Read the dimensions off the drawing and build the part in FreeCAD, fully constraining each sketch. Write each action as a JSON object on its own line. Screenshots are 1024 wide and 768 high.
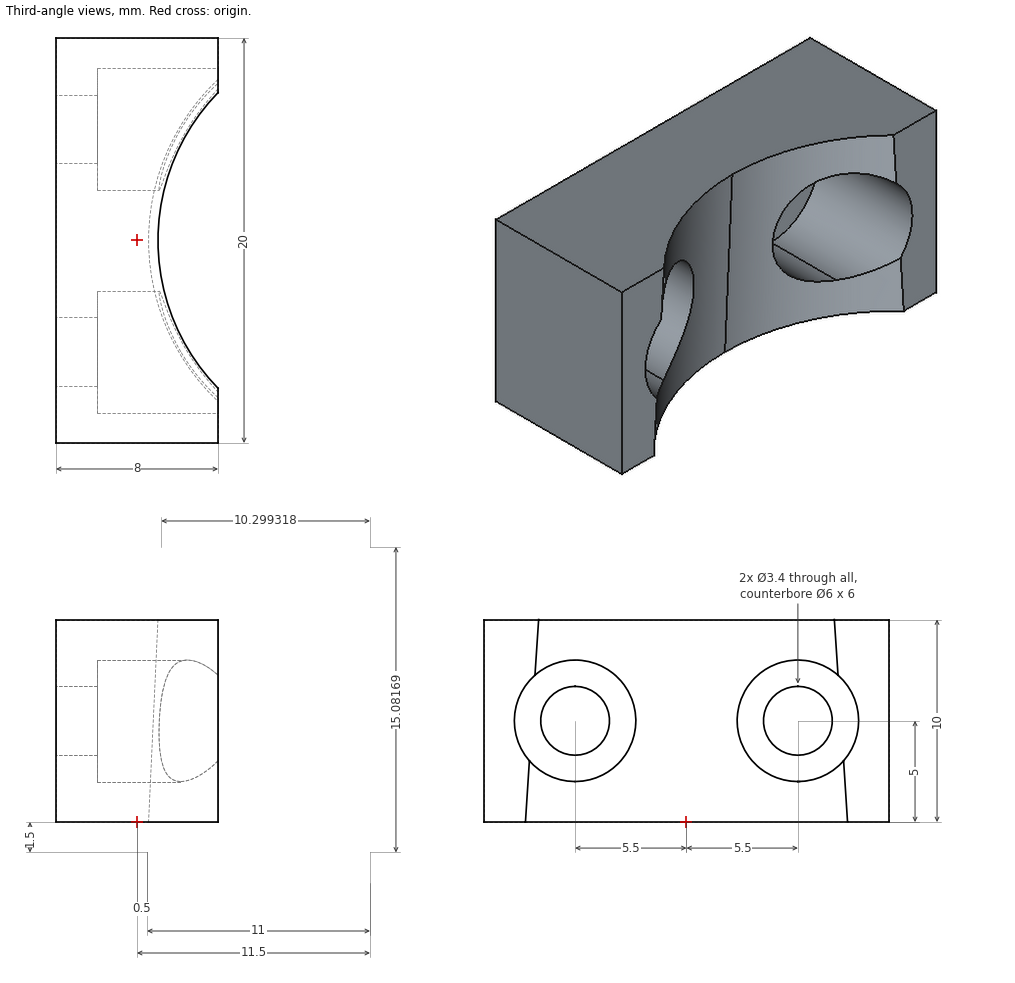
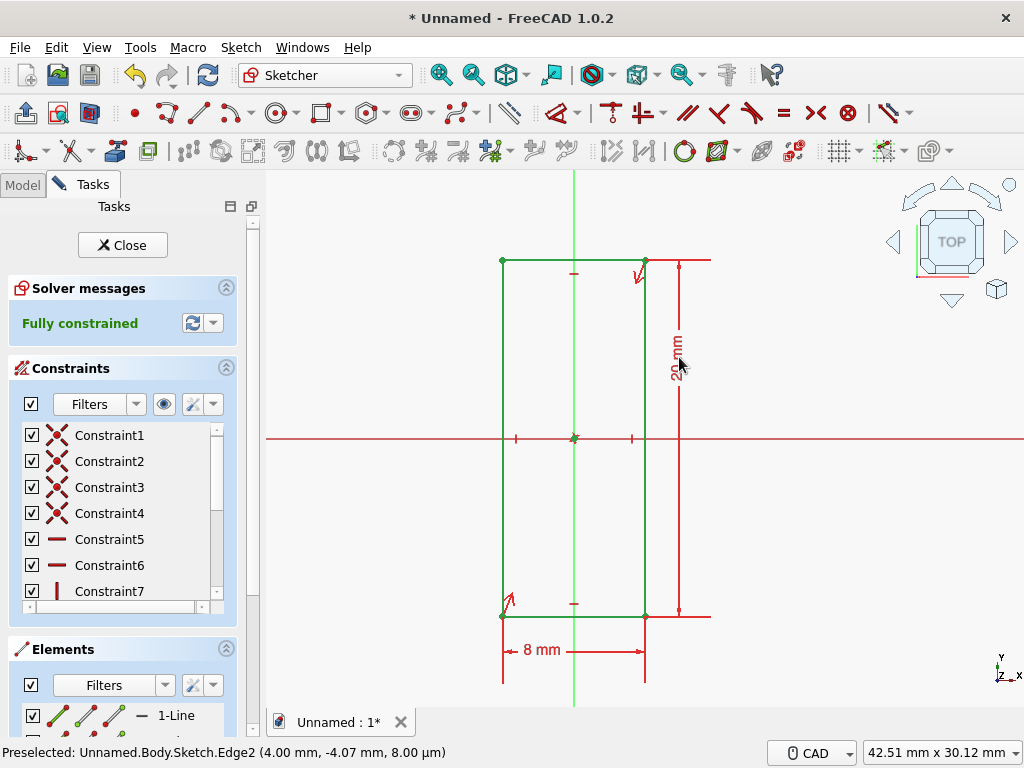
{"action": "left_click", "coordinate": [123, 245]}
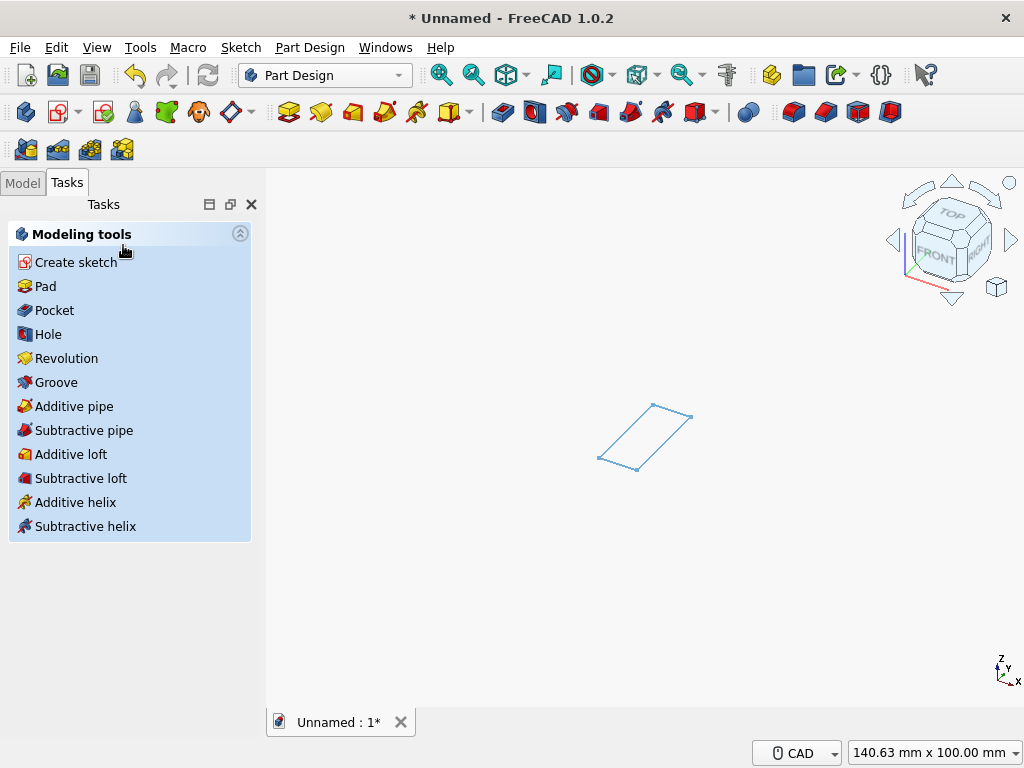
{"action": "left_click", "coordinate": [290, 112]}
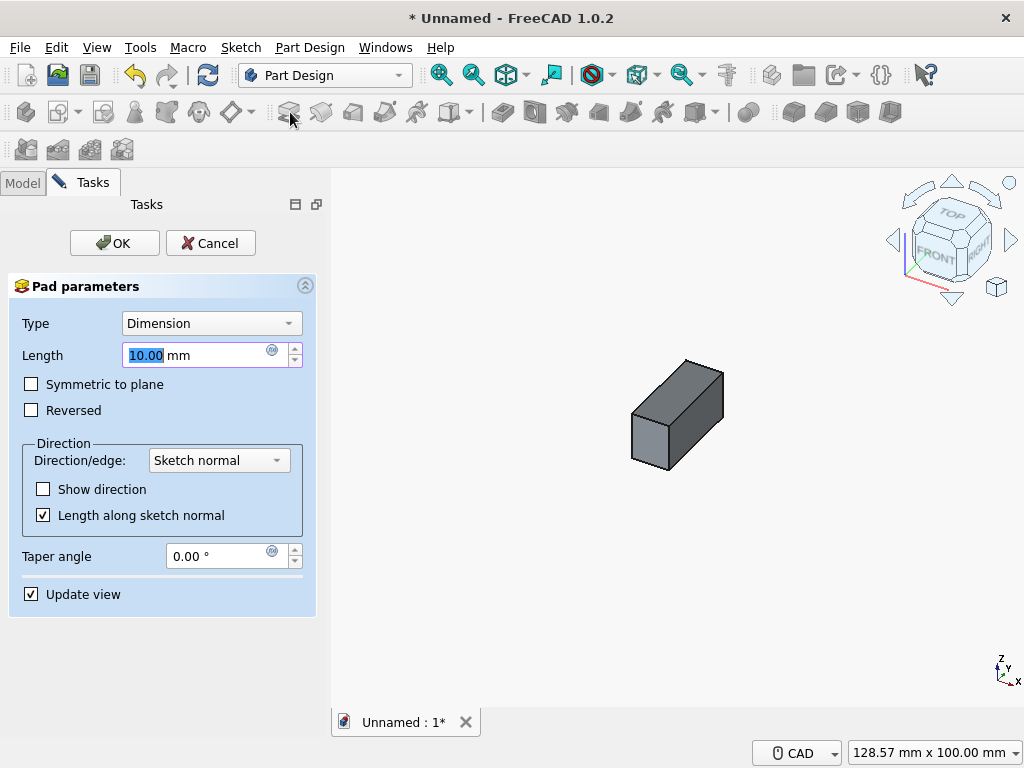
{"action": "type", "text": "10"}
{"action": "key", "text": "Tab"}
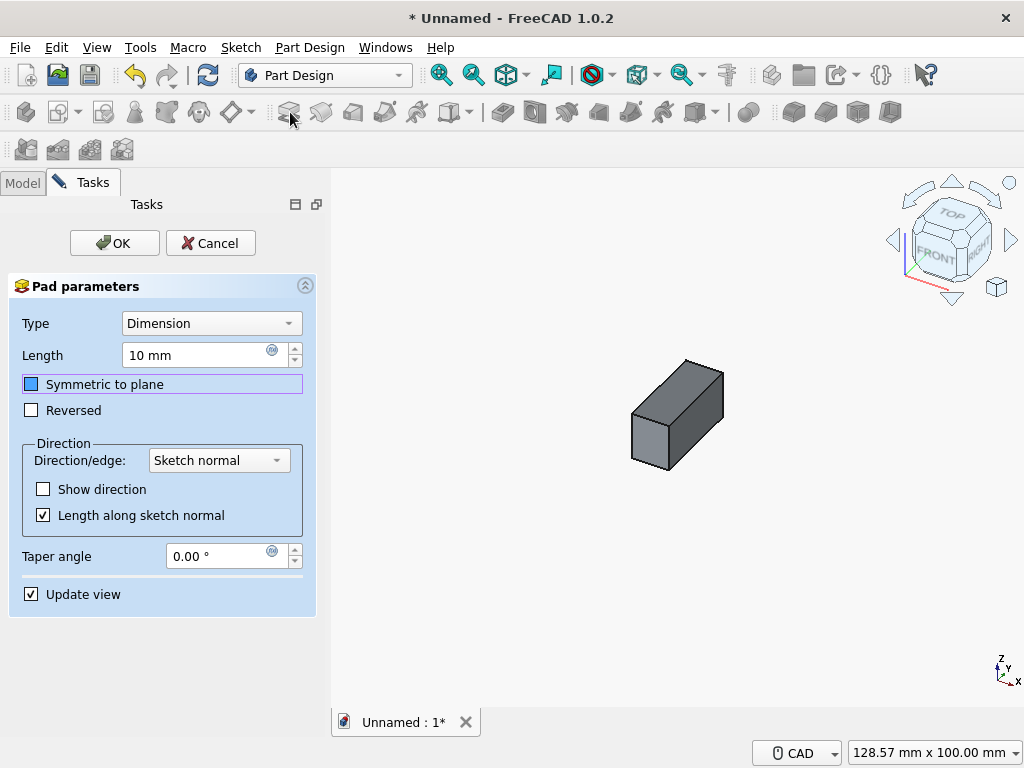
{"action": "left_click", "coordinate": [115, 243]}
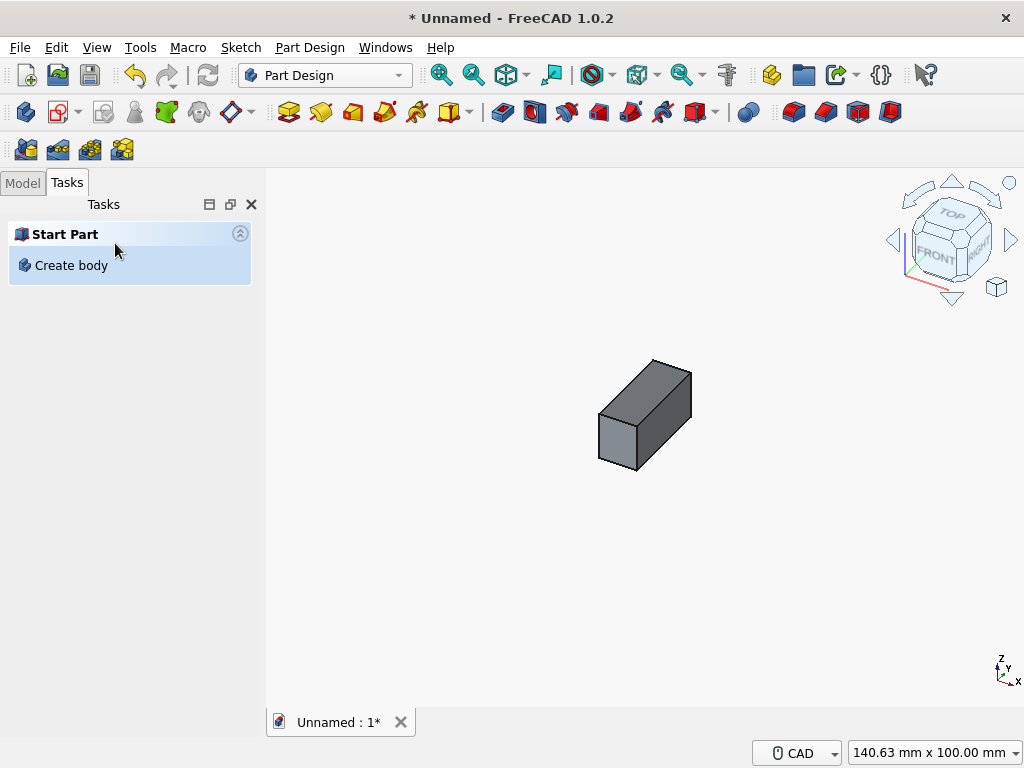
{"action": "key", "text": "v f"}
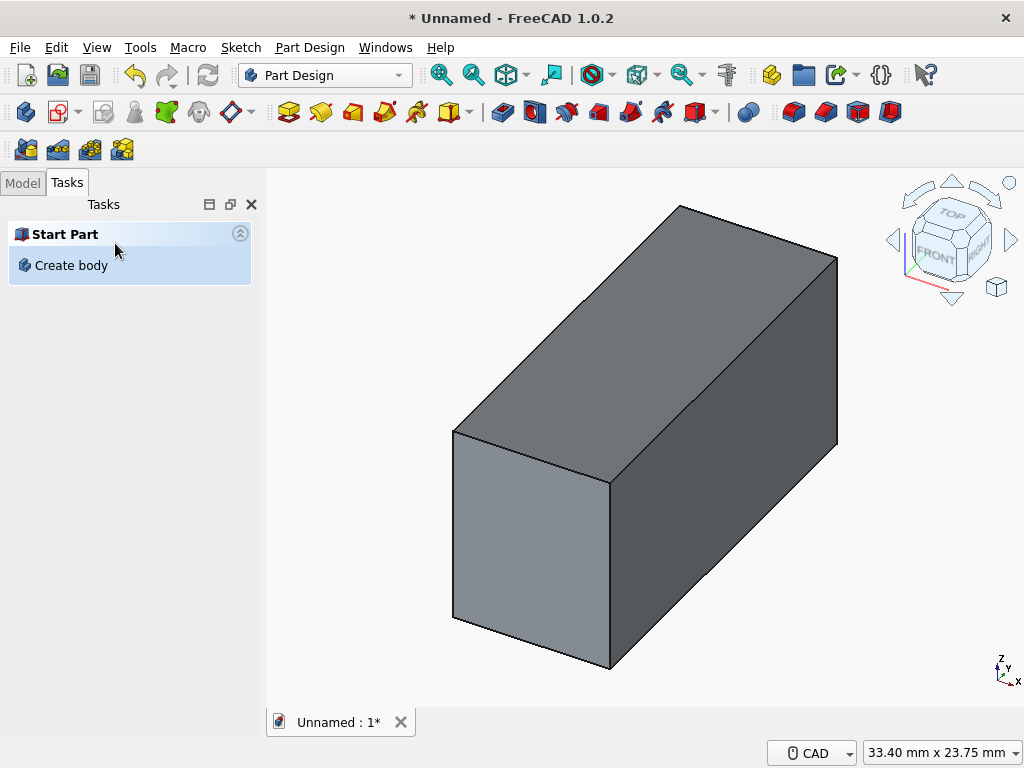
{"action": "left_click", "coordinate": [756, 430]}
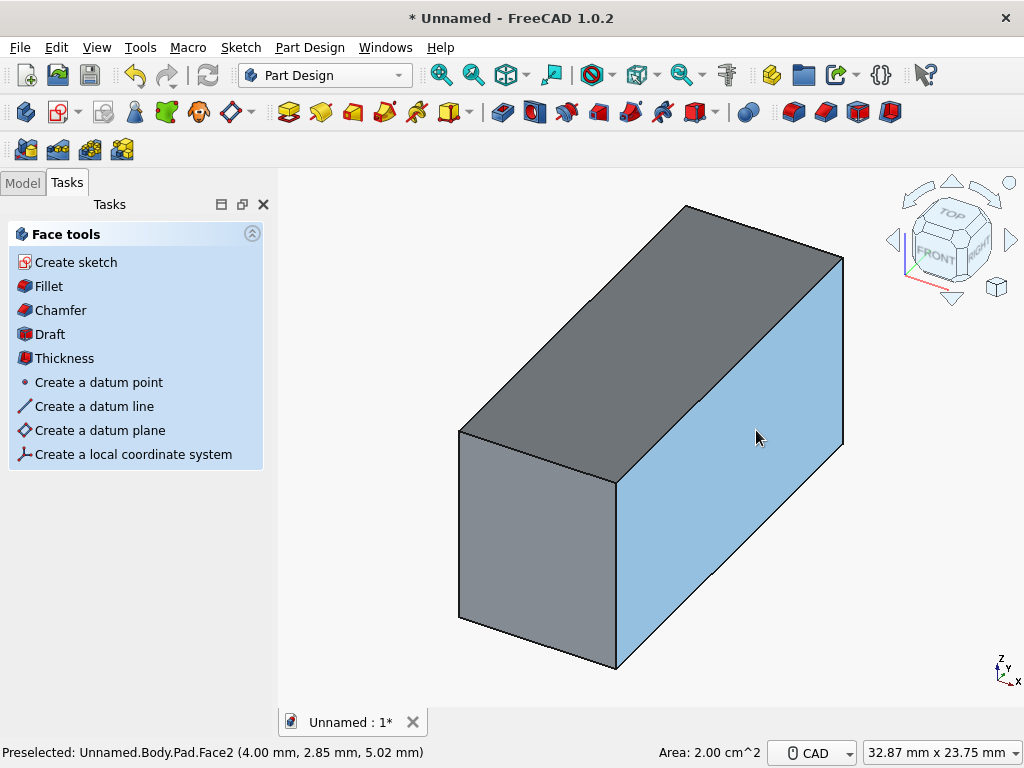
{"action": "left_click", "coordinate": [58, 112]}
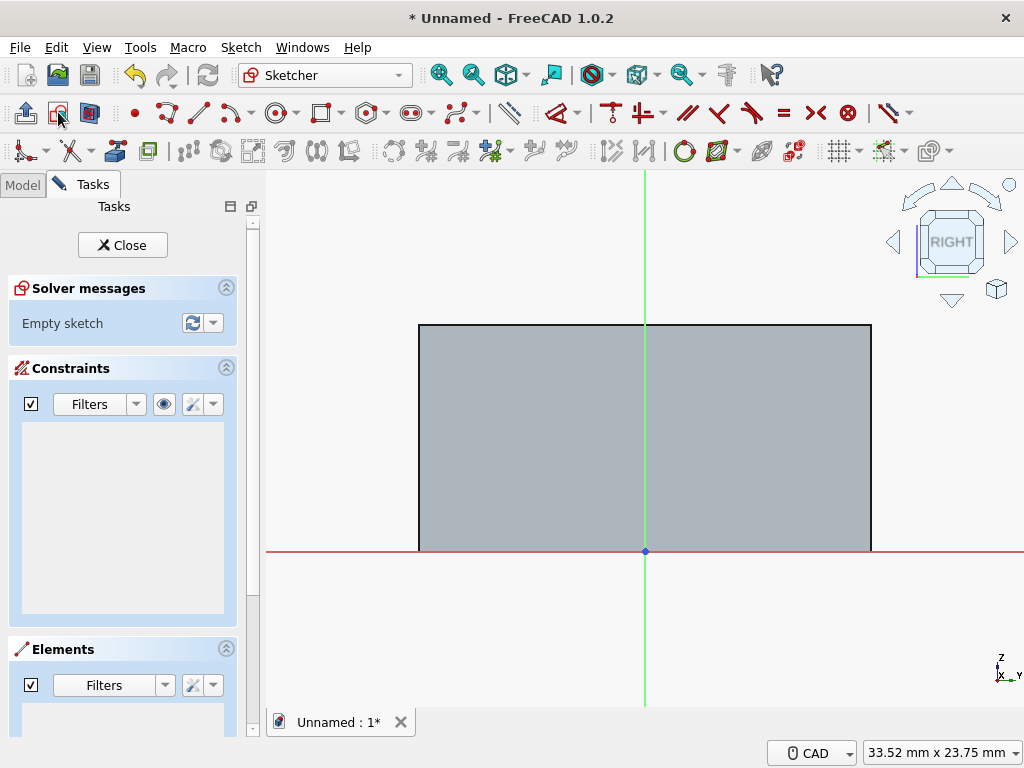
{"action": "left_click", "coordinate": [276, 114]}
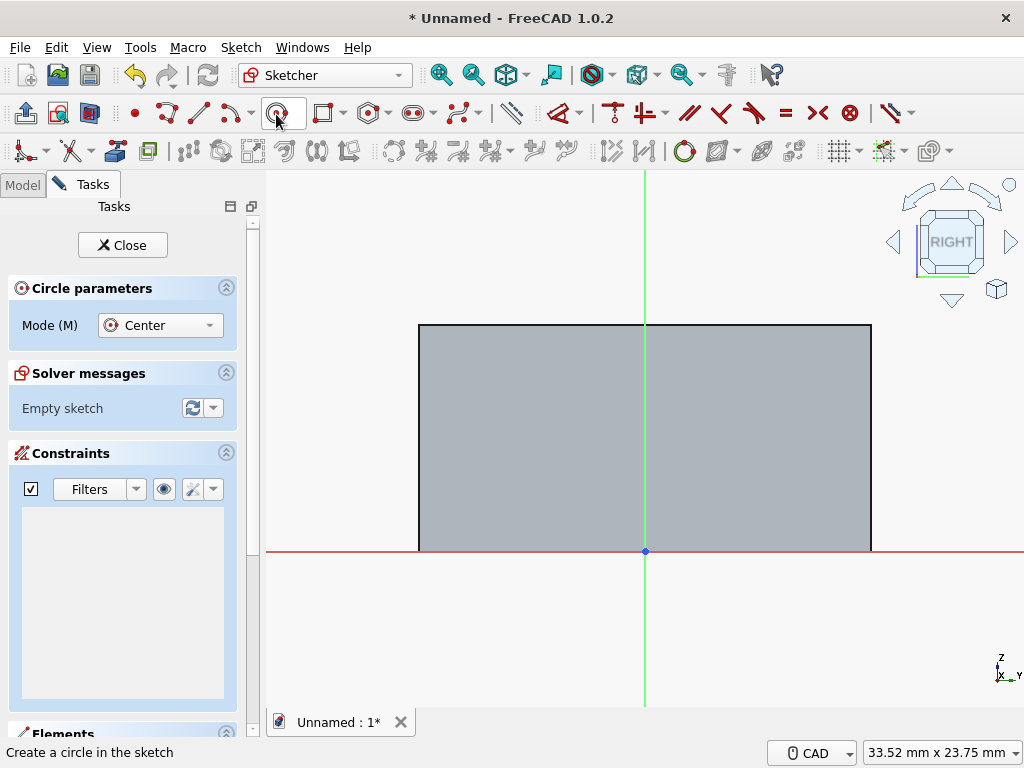
{"action": "left_click", "coordinate": [769, 439]}
{"action": "left_click", "coordinate": [797, 411]}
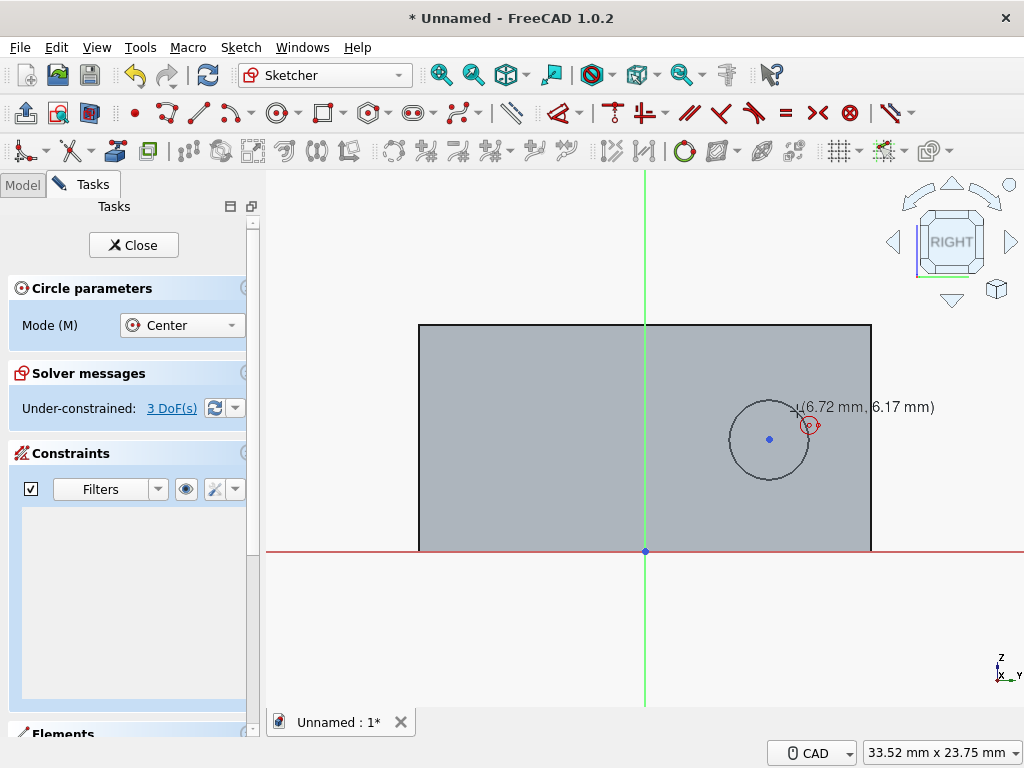
{"action": "left_click", "coordinate": [521, 439]}
{"action": "left_click", "coordinate": [548, 411]}
{"action": "key", "text": "Escape"}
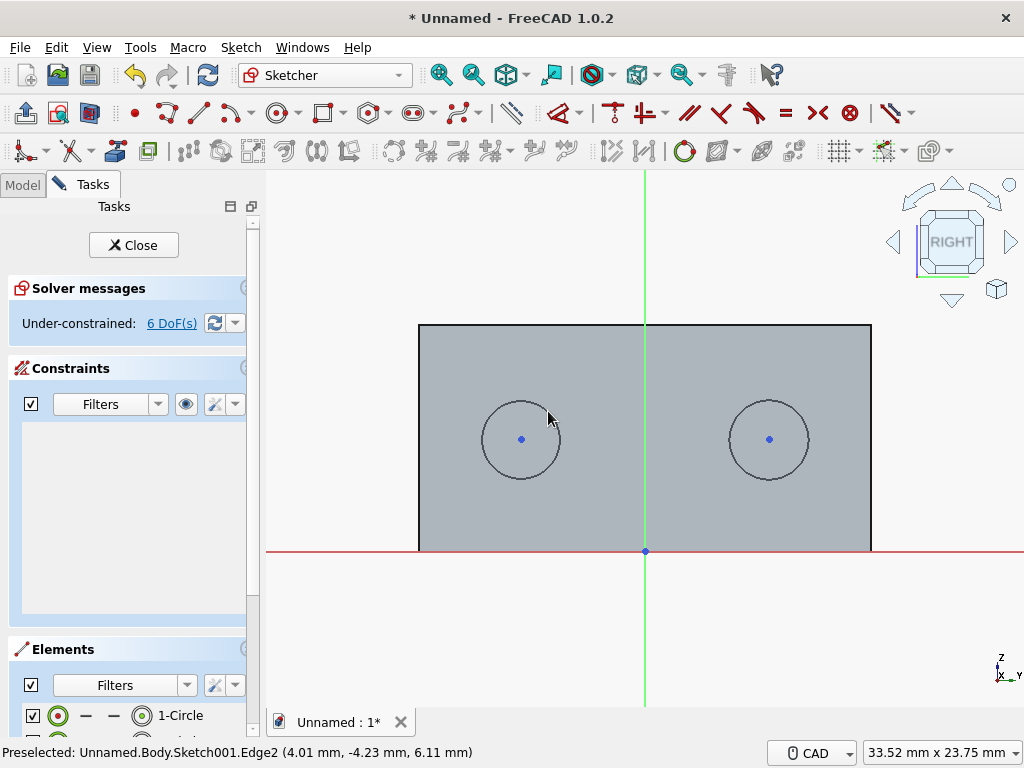
{"action": "left_click", "coordinate": [797, 412]}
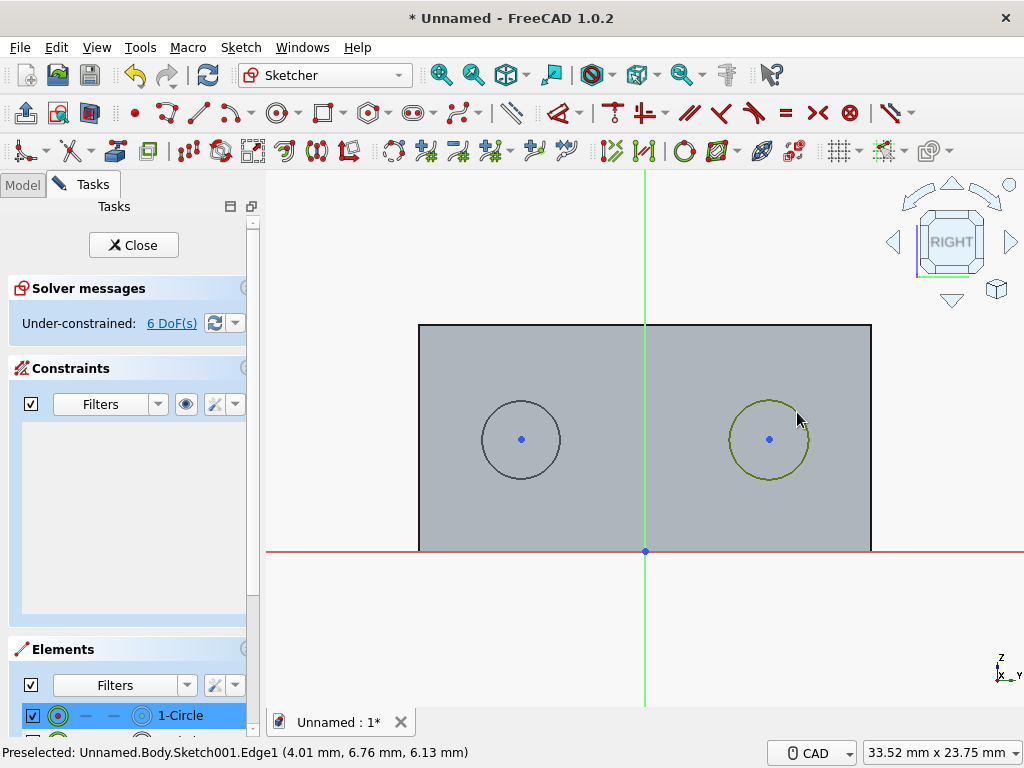
{"action": "left_click", "coordinate": [548, 412]}